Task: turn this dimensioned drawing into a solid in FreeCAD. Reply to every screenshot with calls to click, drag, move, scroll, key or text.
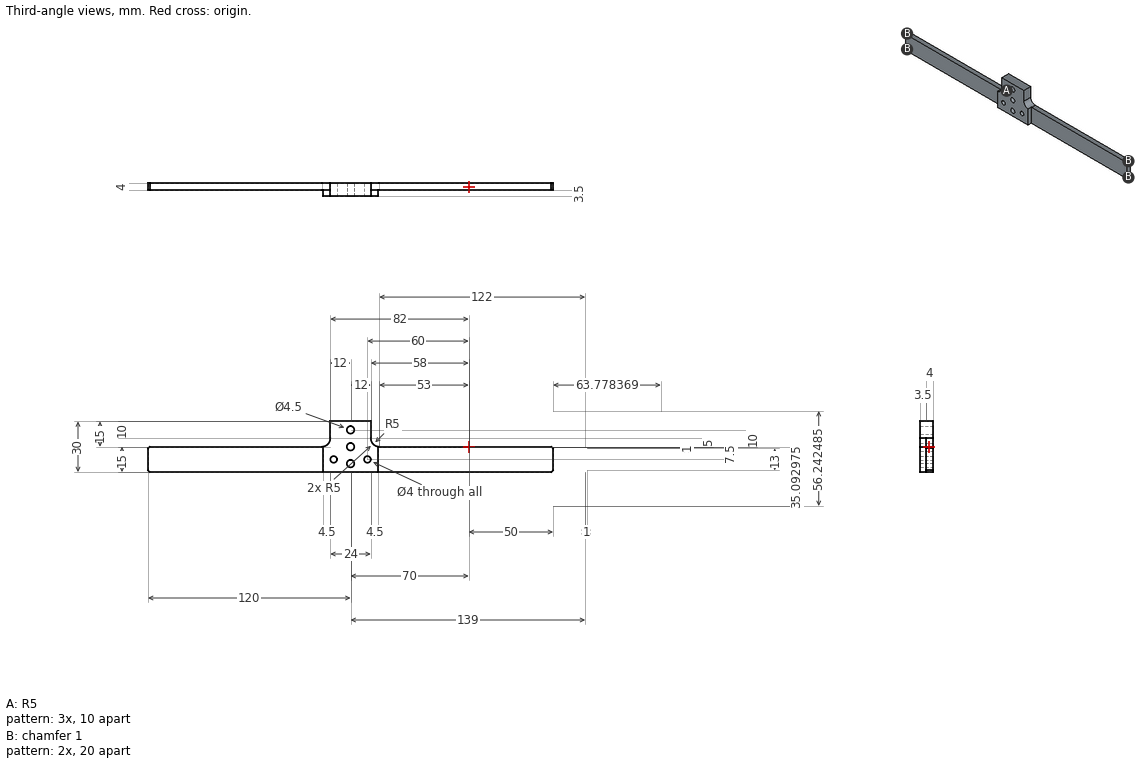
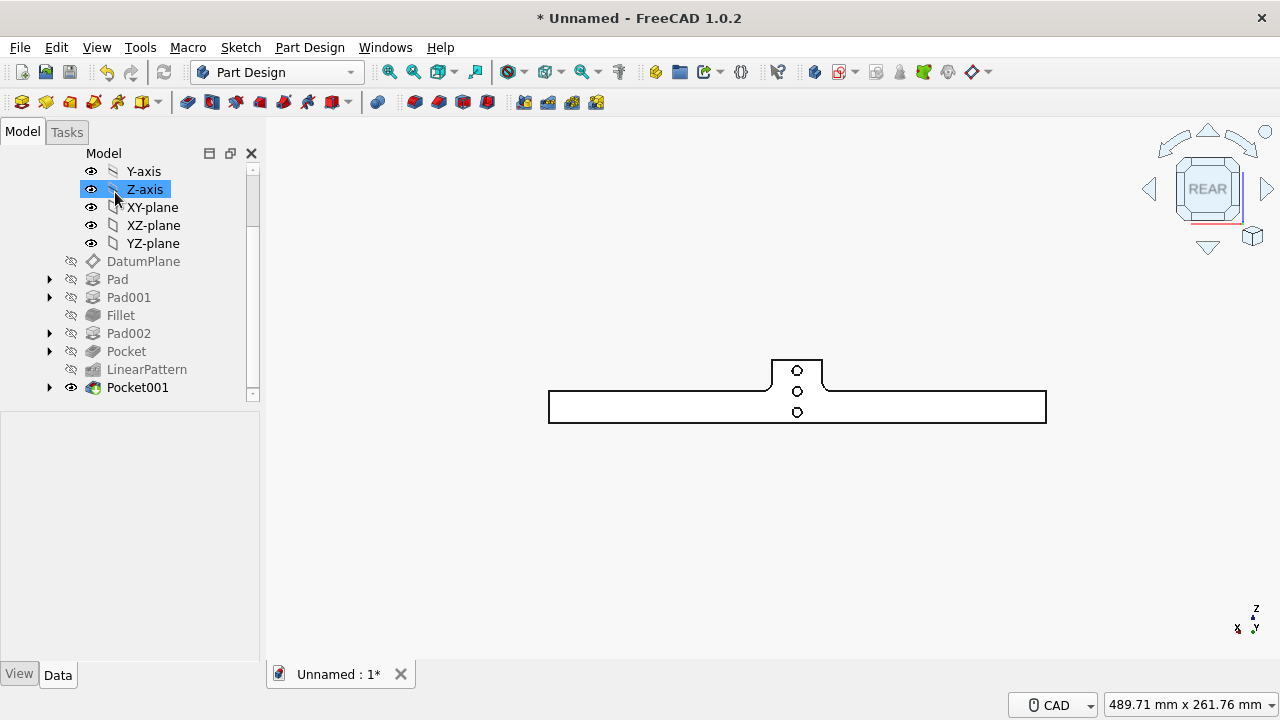
scroll(549, 422, up, 8)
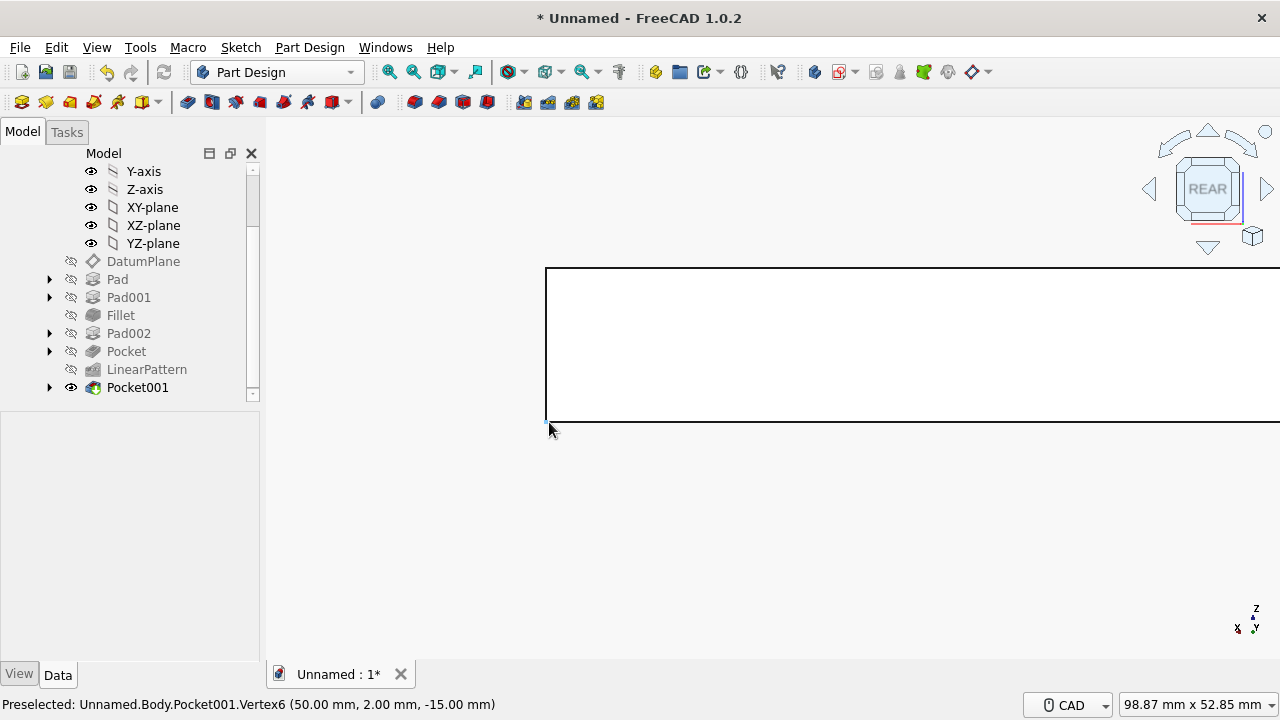
click(390, 72)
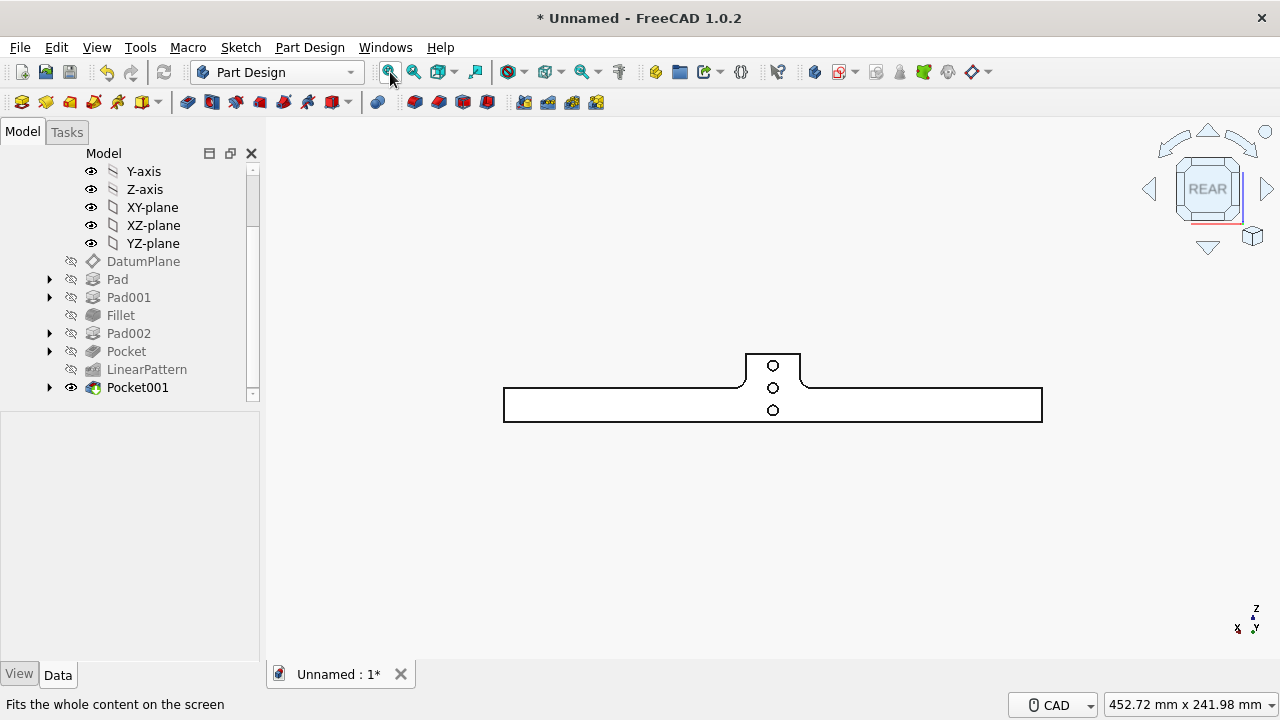
key(0)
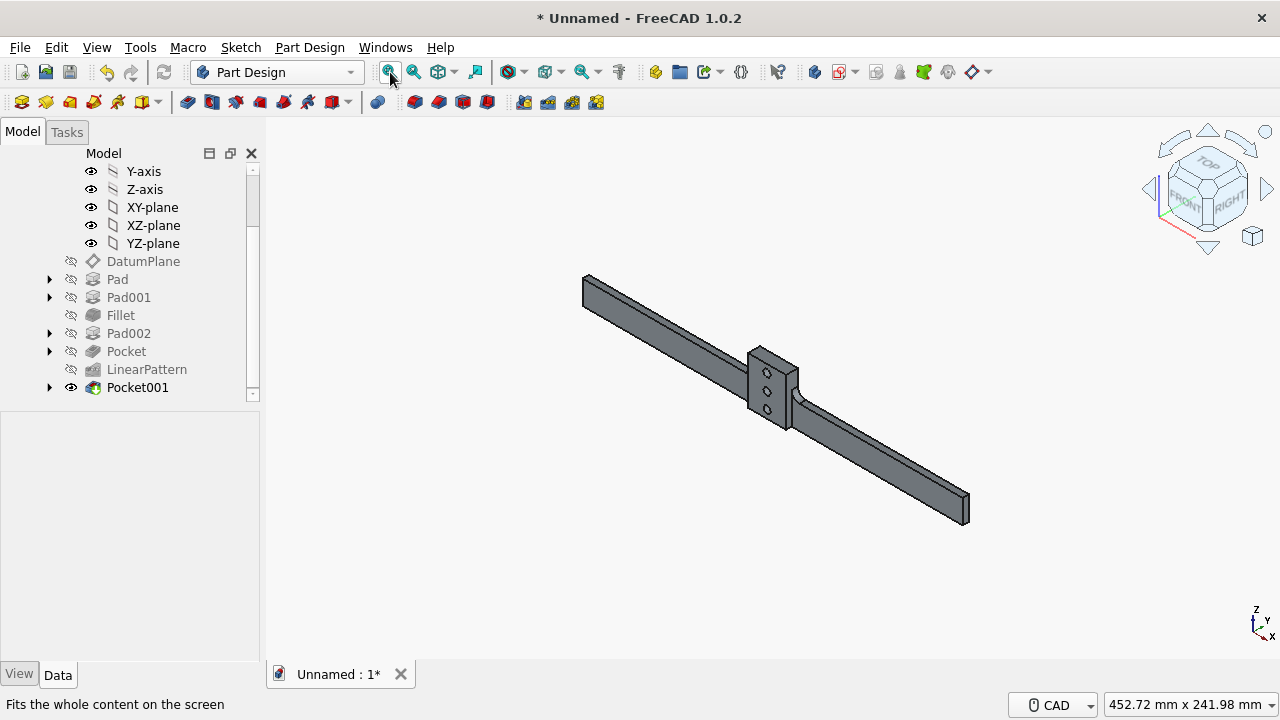
scroll(966, 523, up, 8)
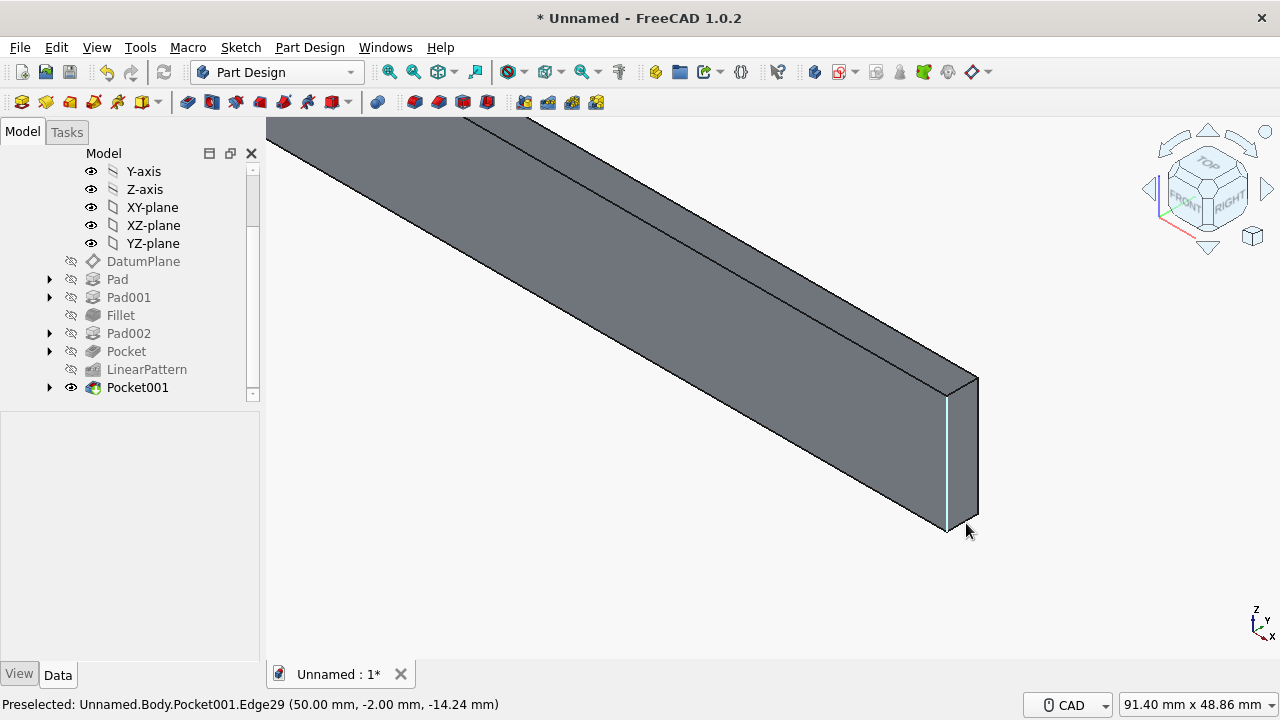
click(962, 386)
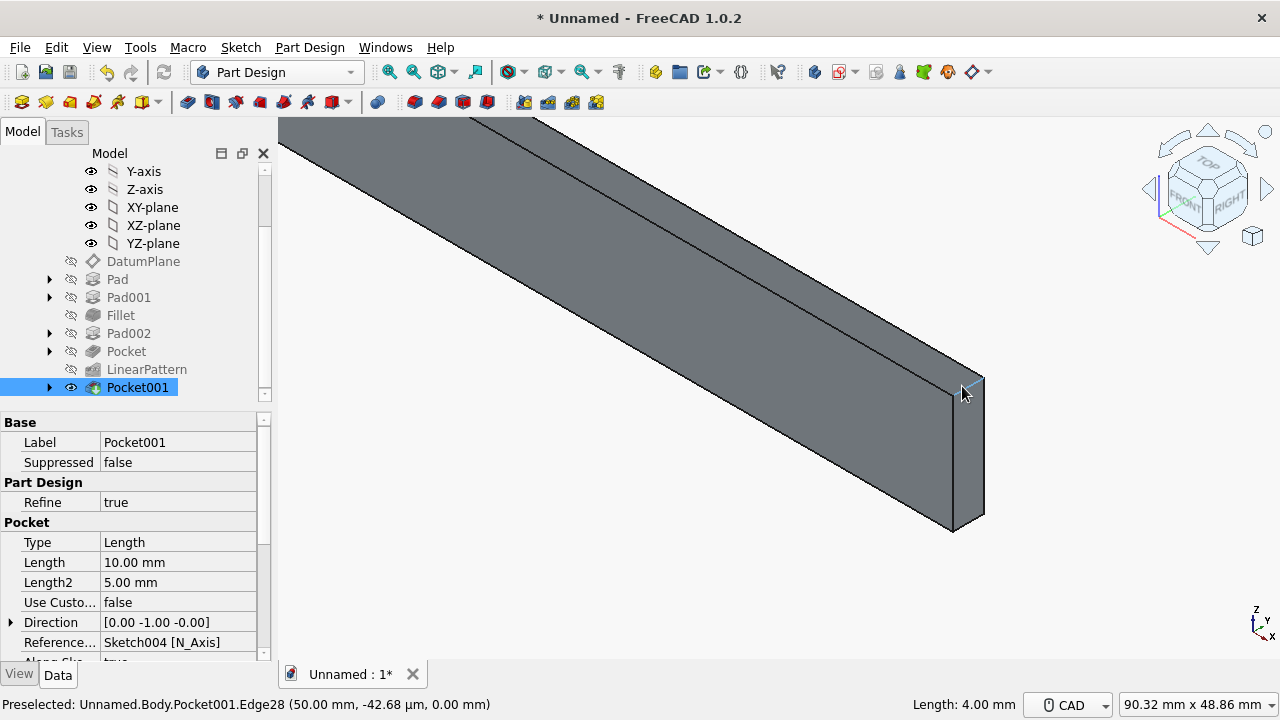
click(390, 72)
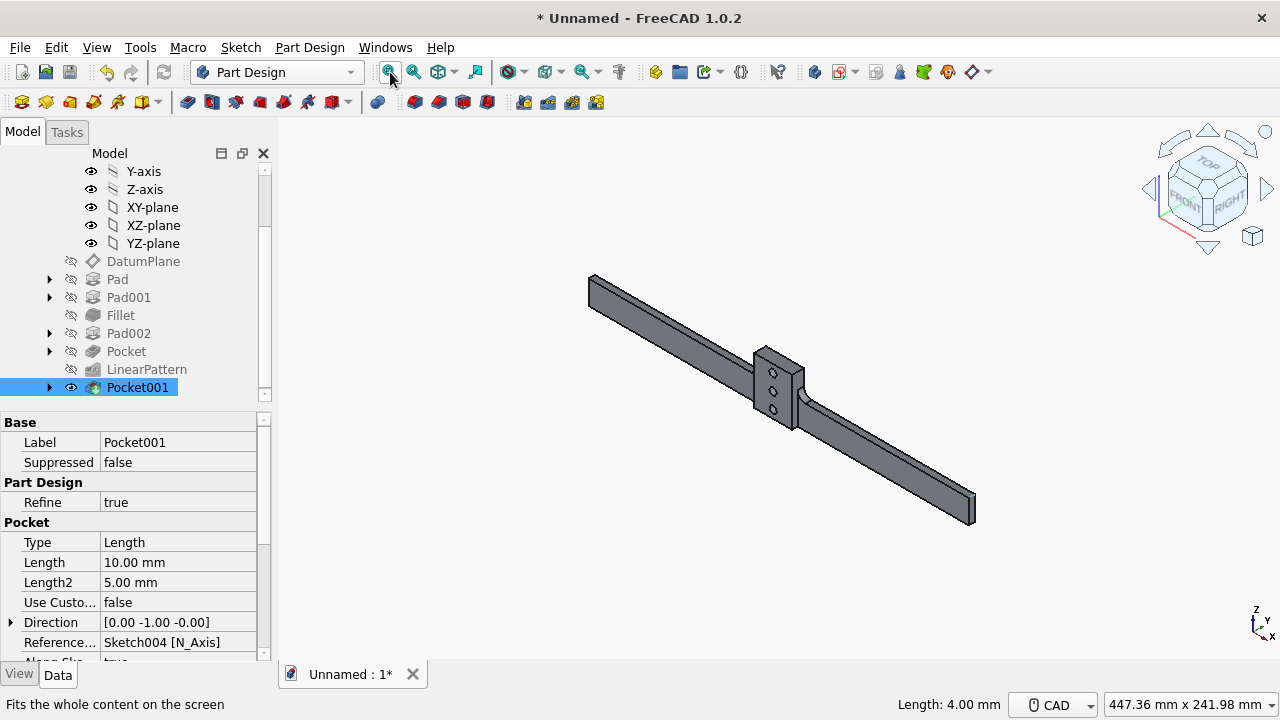
key(2)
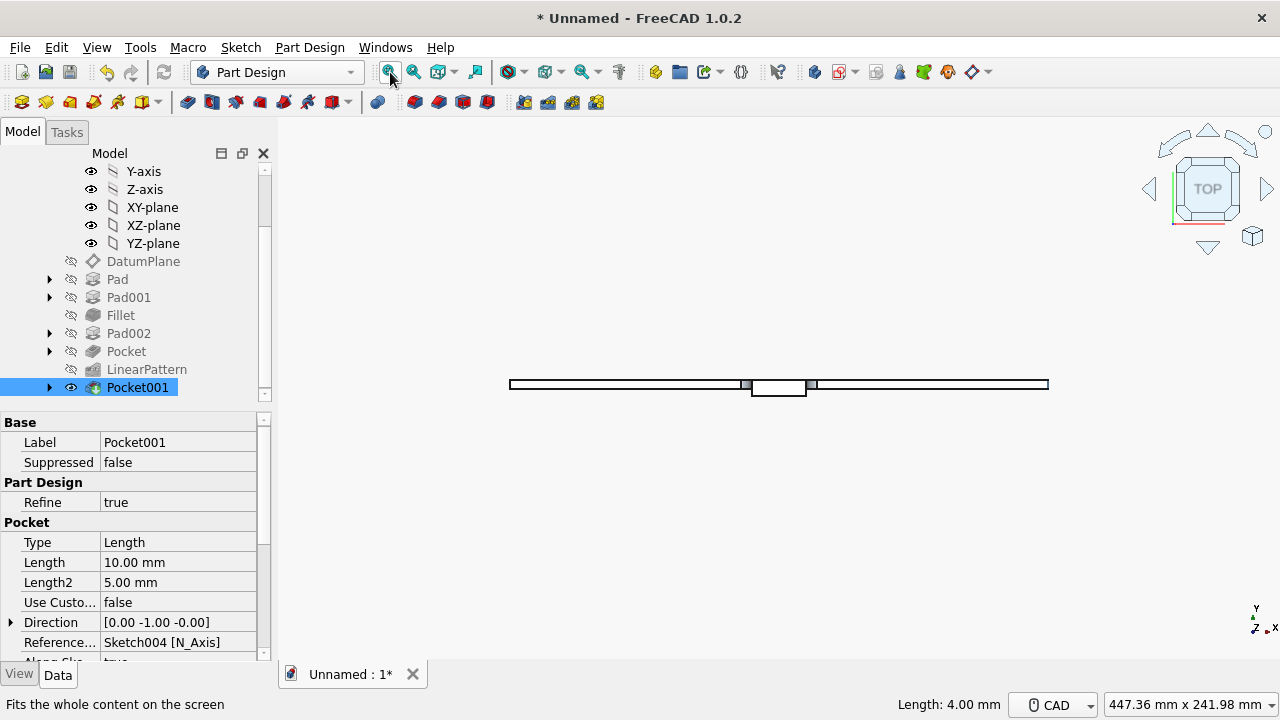
click(510, 385, ctrl)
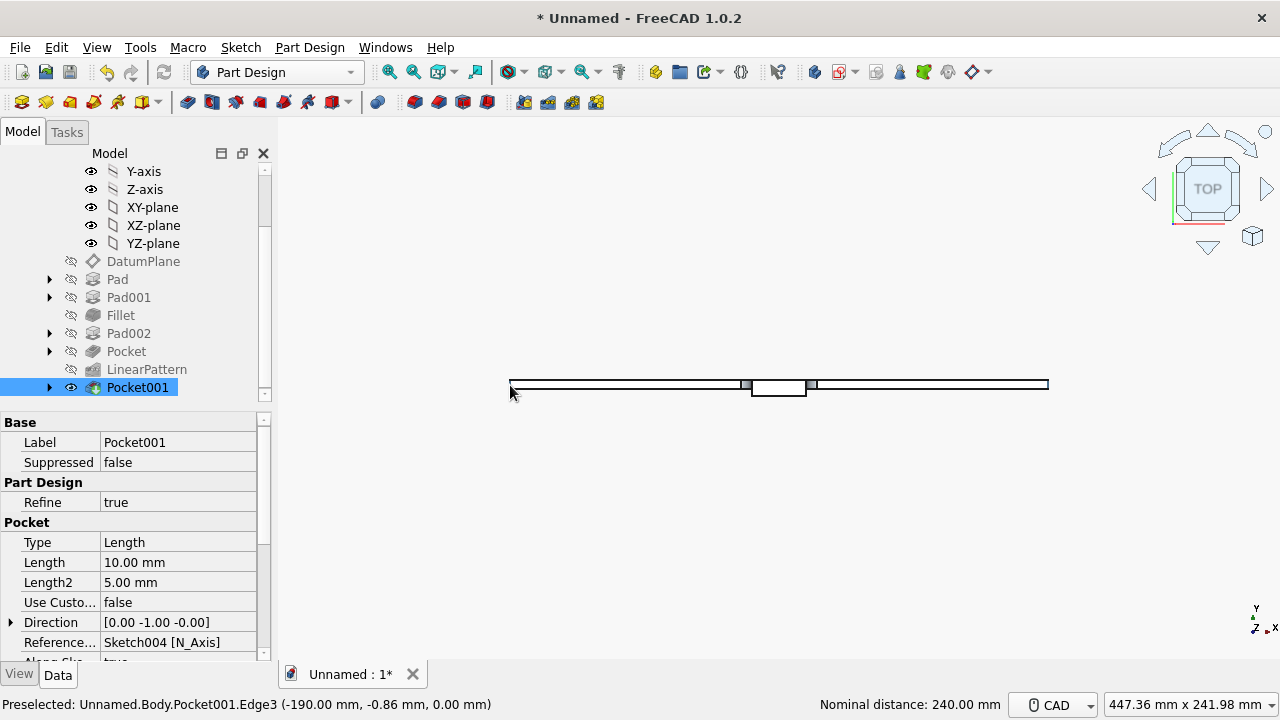
scroll(1048, 383, up, 8)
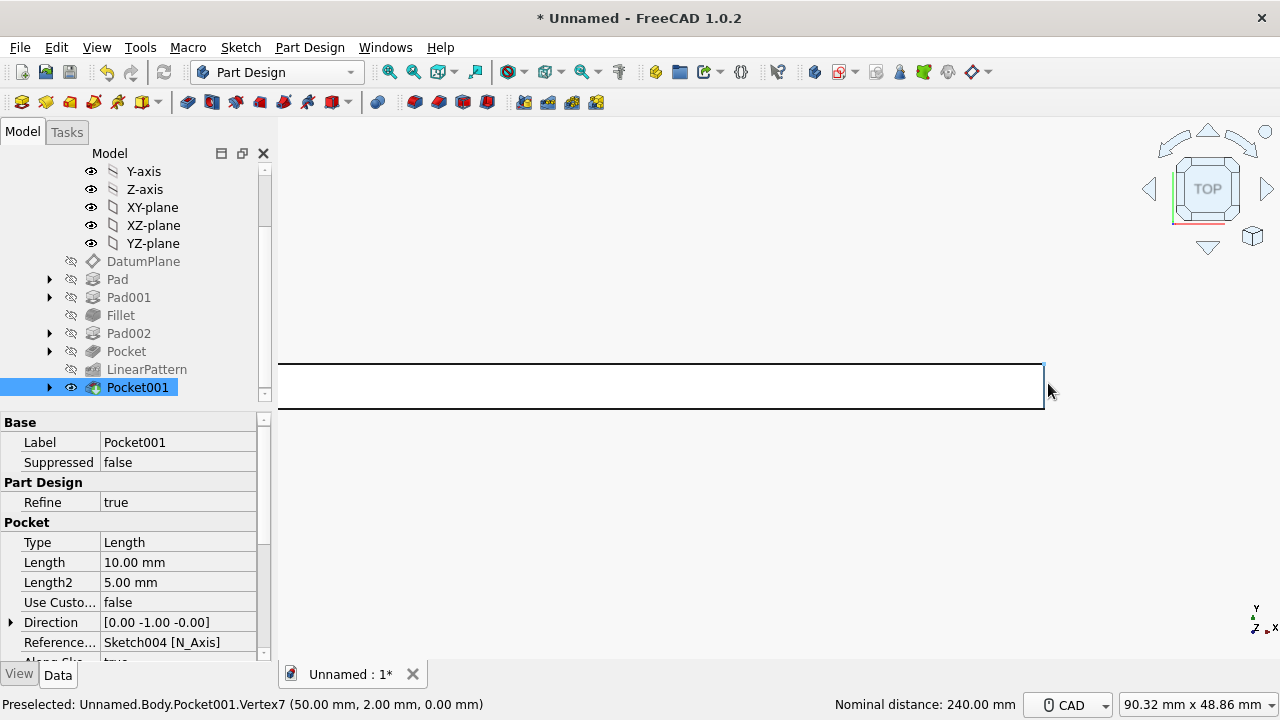
click(390, 72)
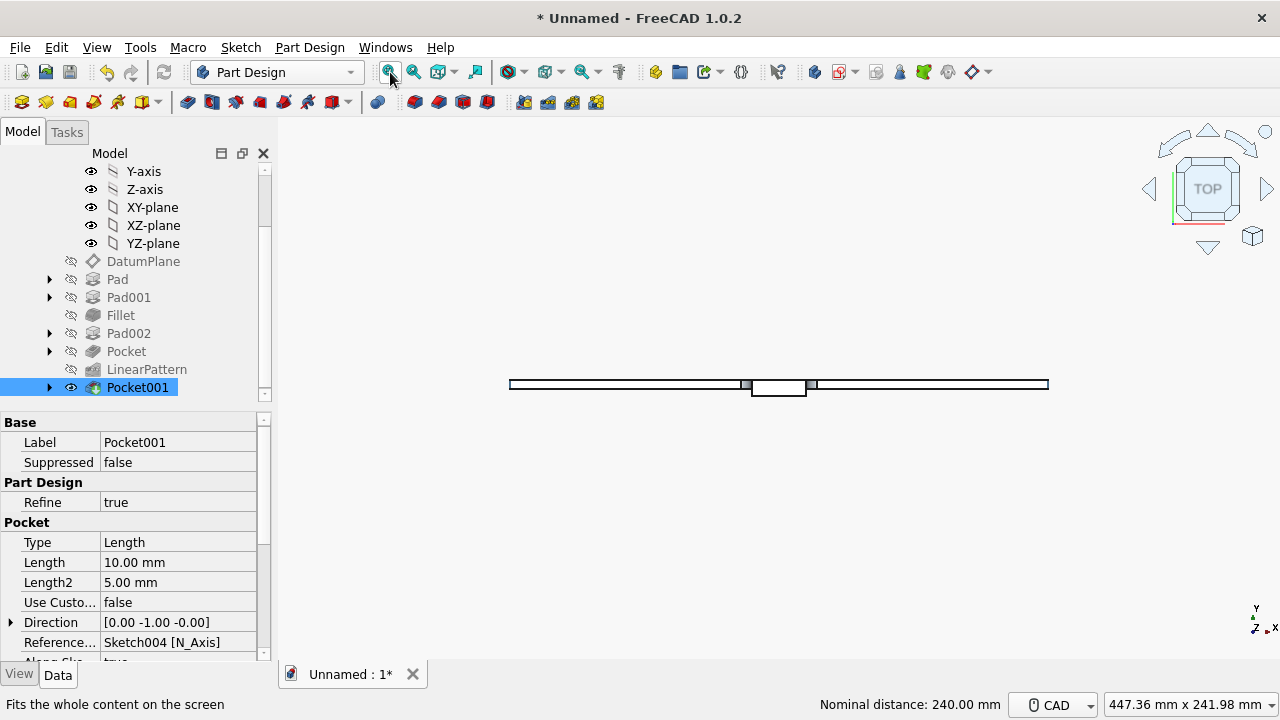
key(1)